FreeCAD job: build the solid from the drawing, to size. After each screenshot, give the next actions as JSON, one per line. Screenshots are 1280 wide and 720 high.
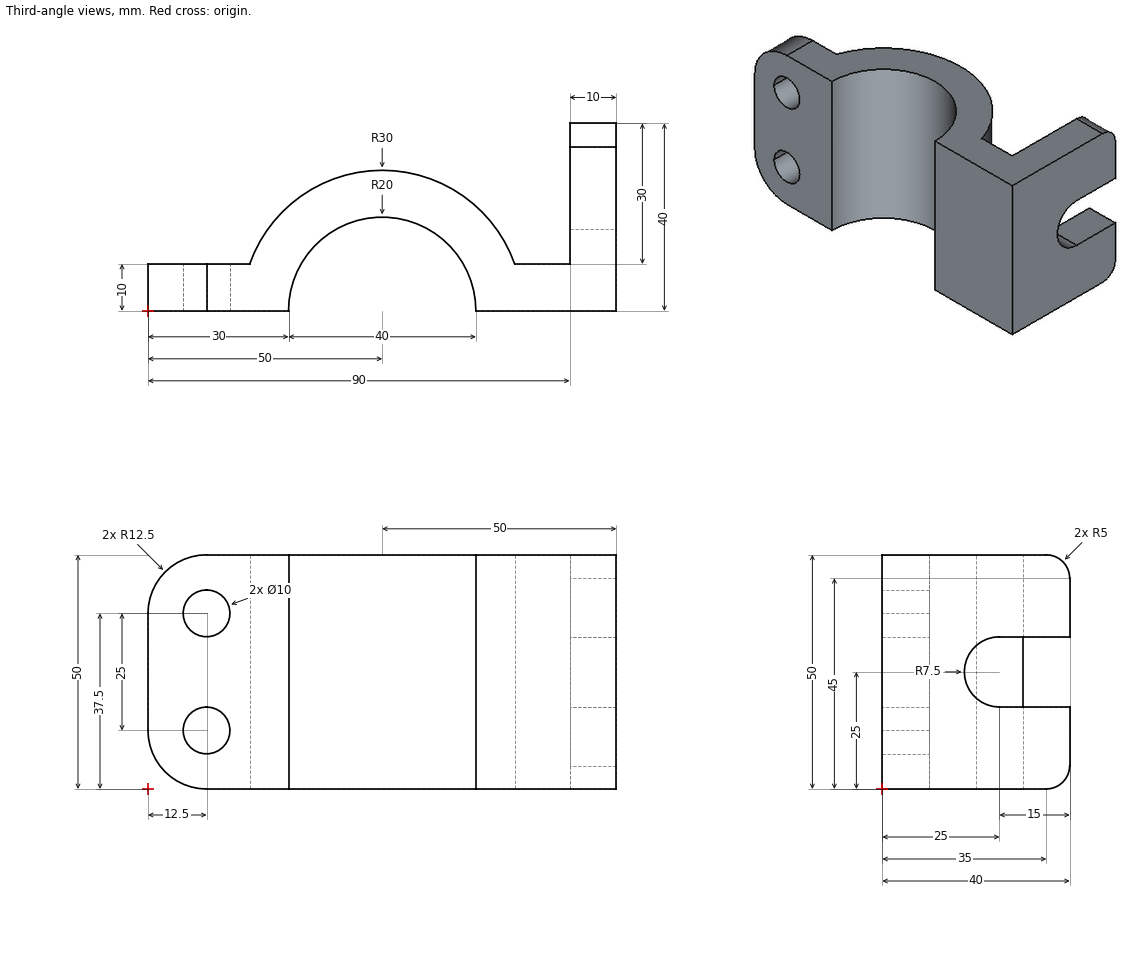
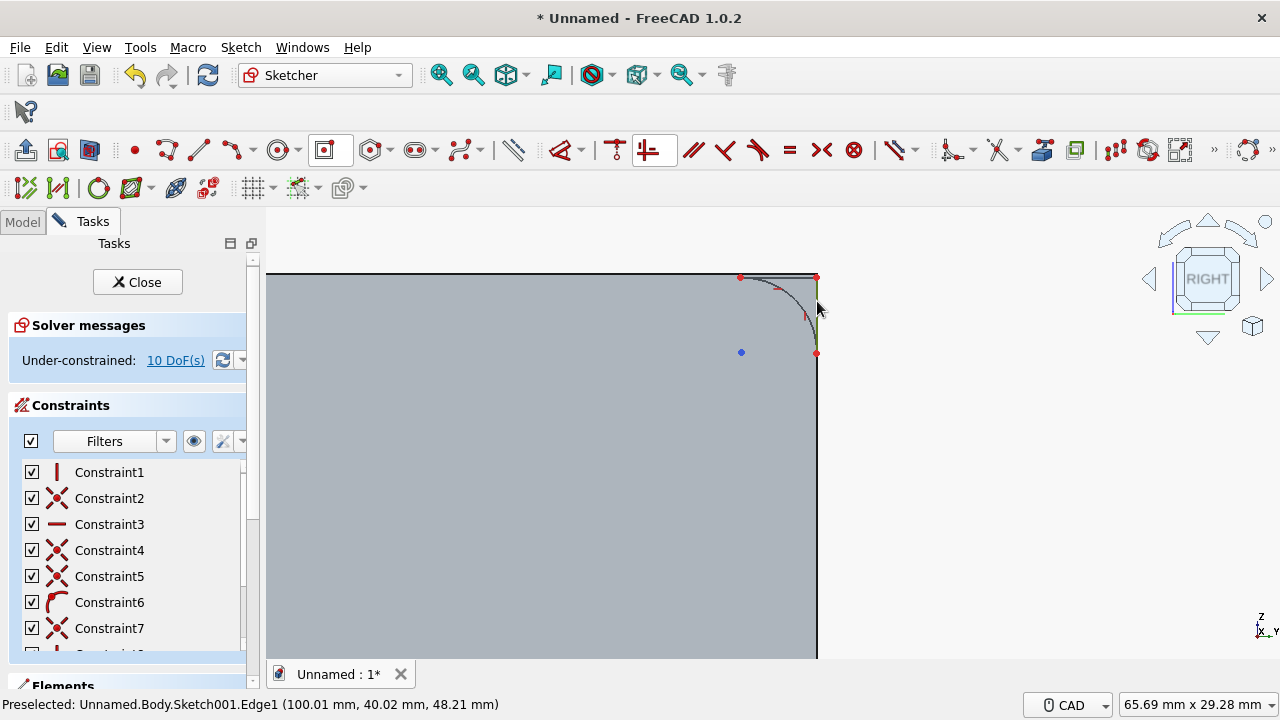
{"action": "left_click", "coordinate": [795, 300]}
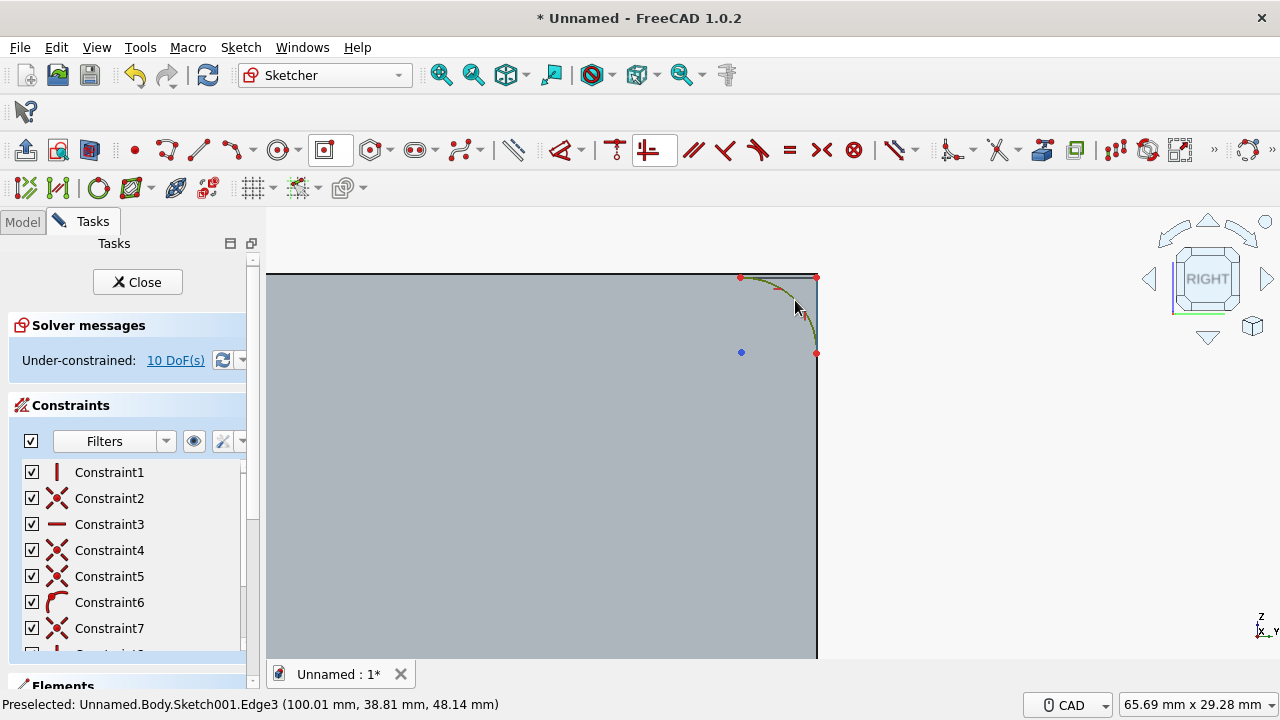
{"action": "left_click", "coordinate": [758, 150]}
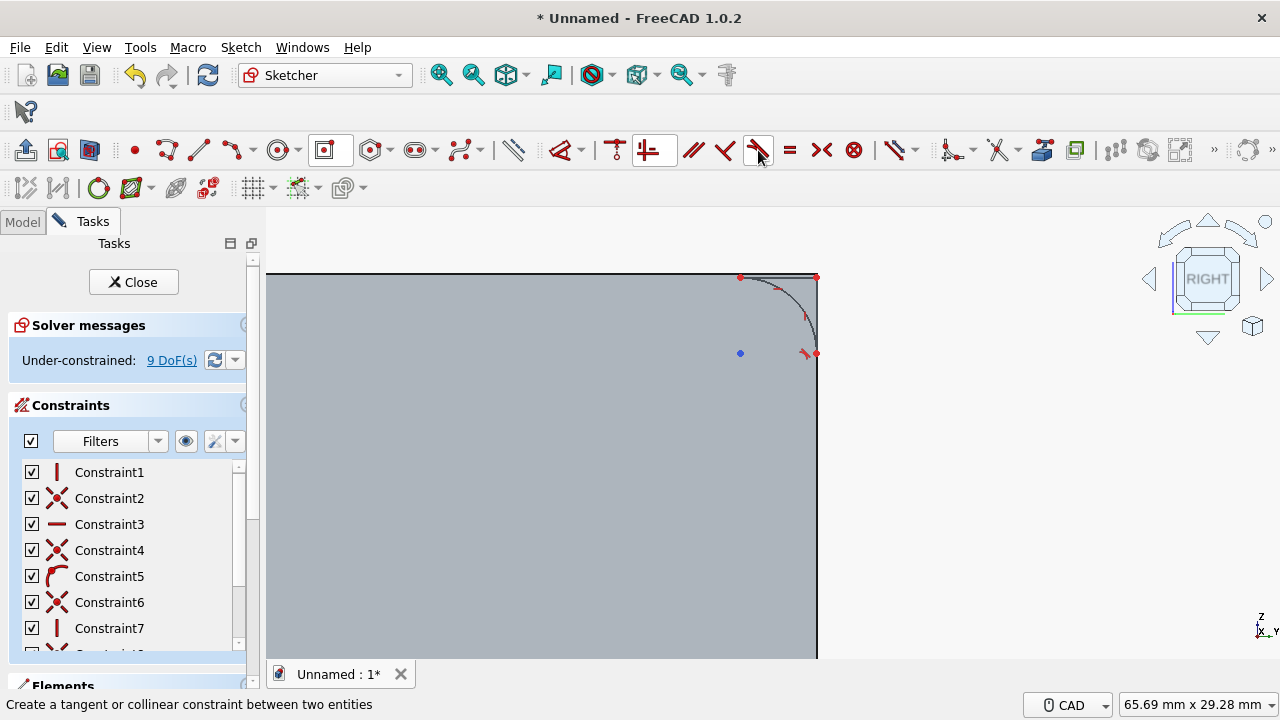
{"action": "left_click", "coordinate": [794, 278]}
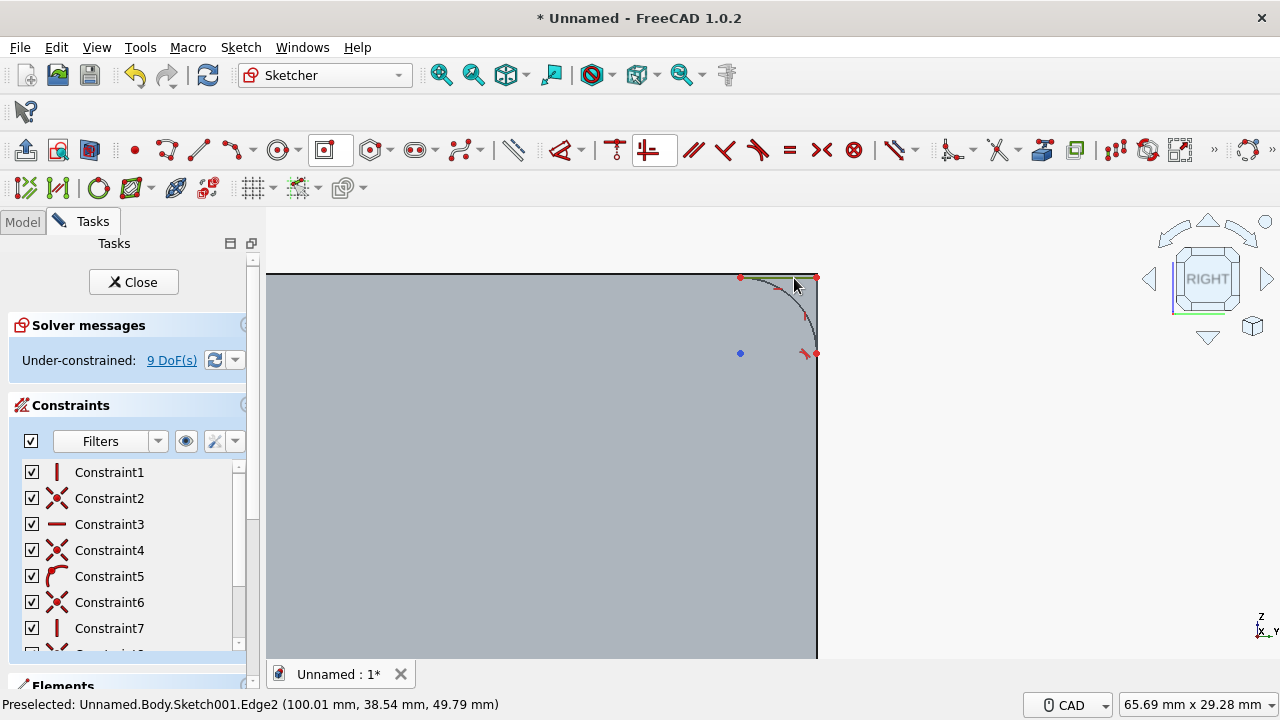
{"action": "left_click", "coordinate": [795, 300]}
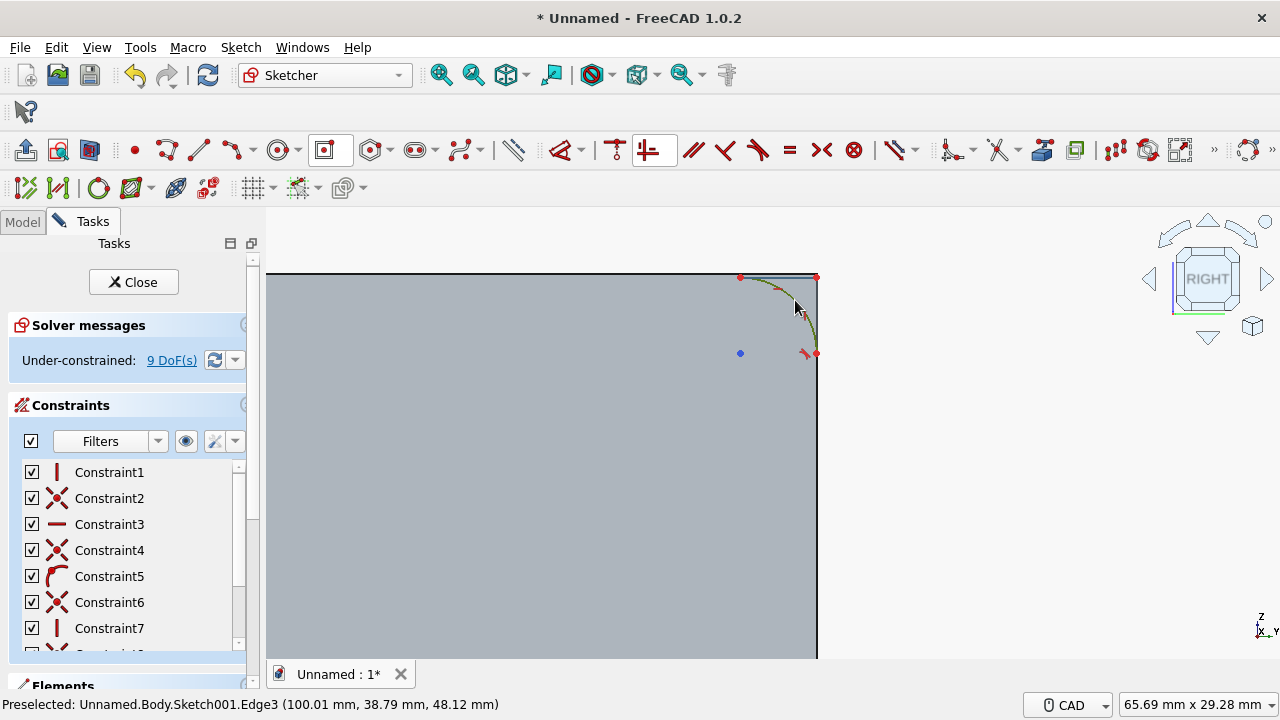
{"action": "left_click", "coordinate": [758, 150]}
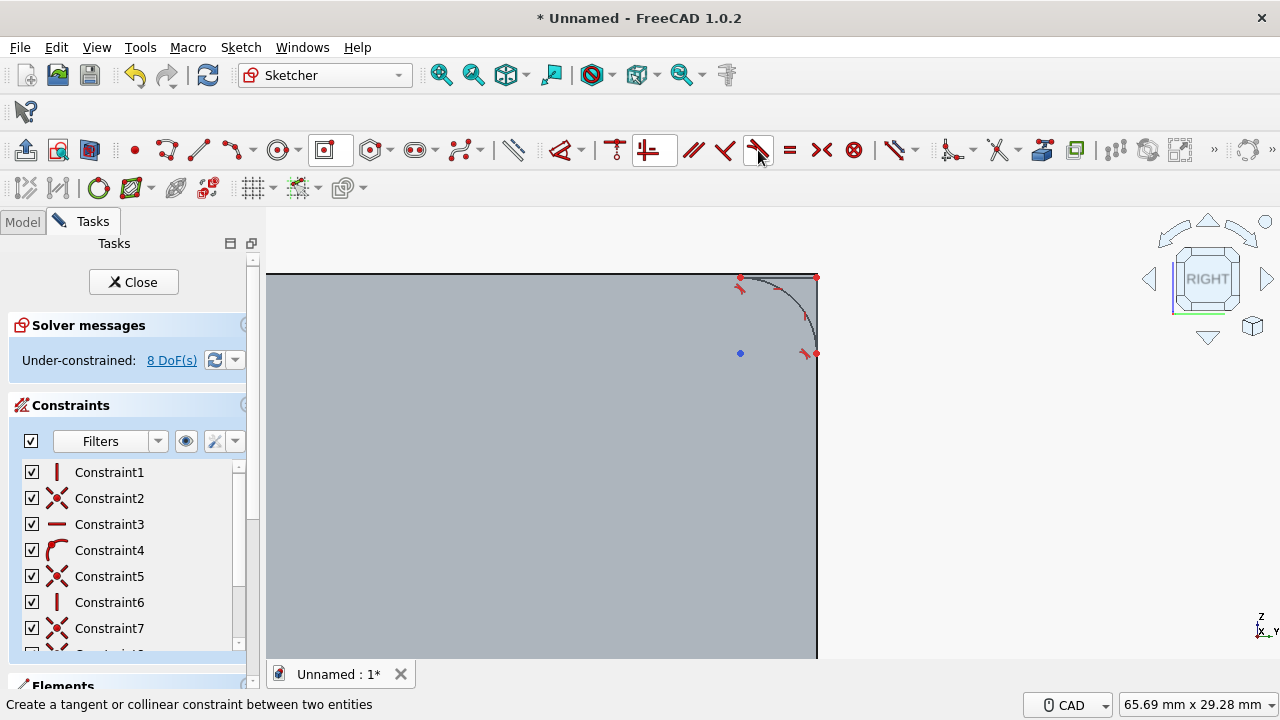
{"action": "scroll", "coordinate": [819, 301], "scroll_direction": "down", "scroll_amount": 5}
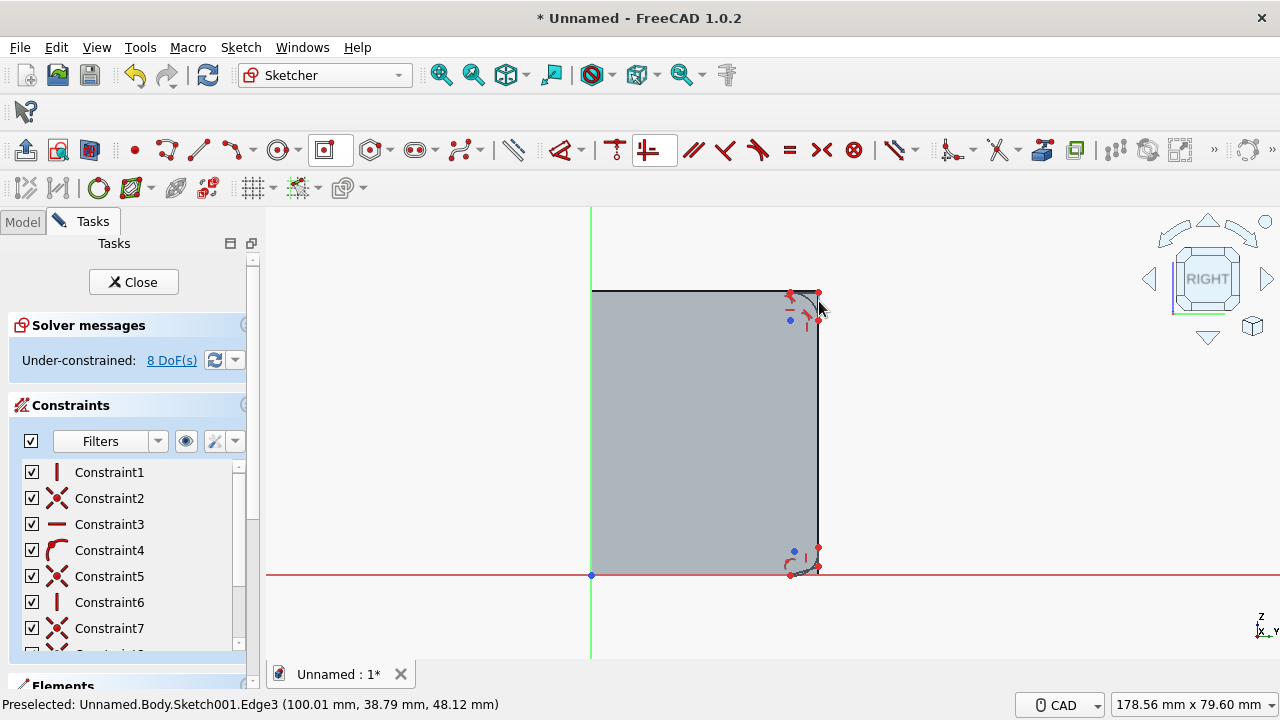
{"action": "scroll", "coordinate": [801, 572], "scroll_direction": "up", "scroll_amount": 9}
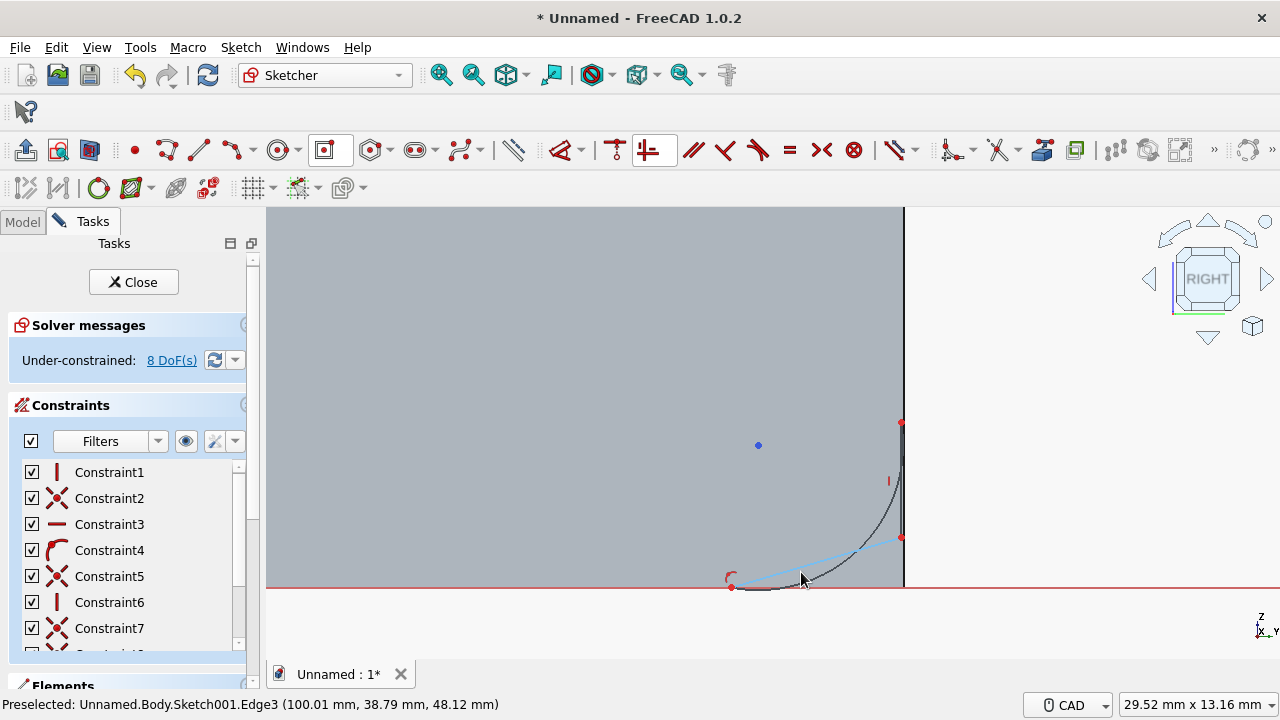
{"action": "left_click", "coordinate": [800, 568]}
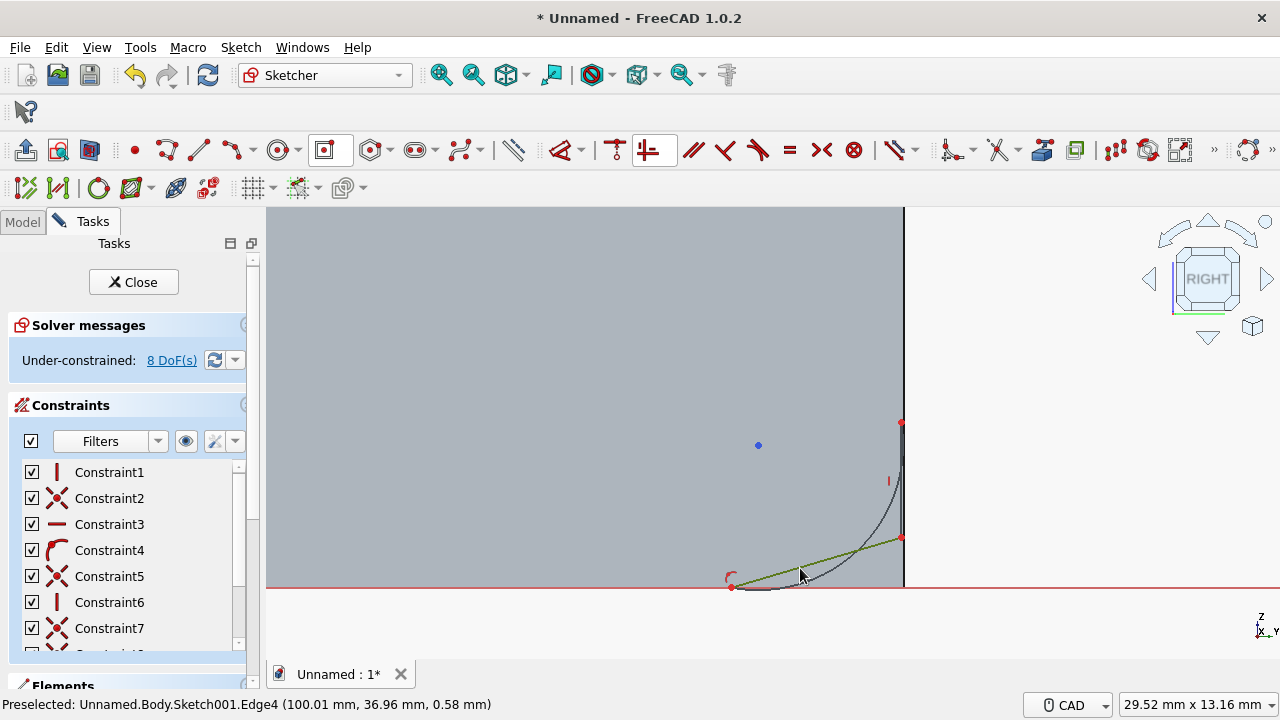
{"action": "scroll", "coordinate": [891, 504], "scroll_direction": "up", "scroll_amount": 2}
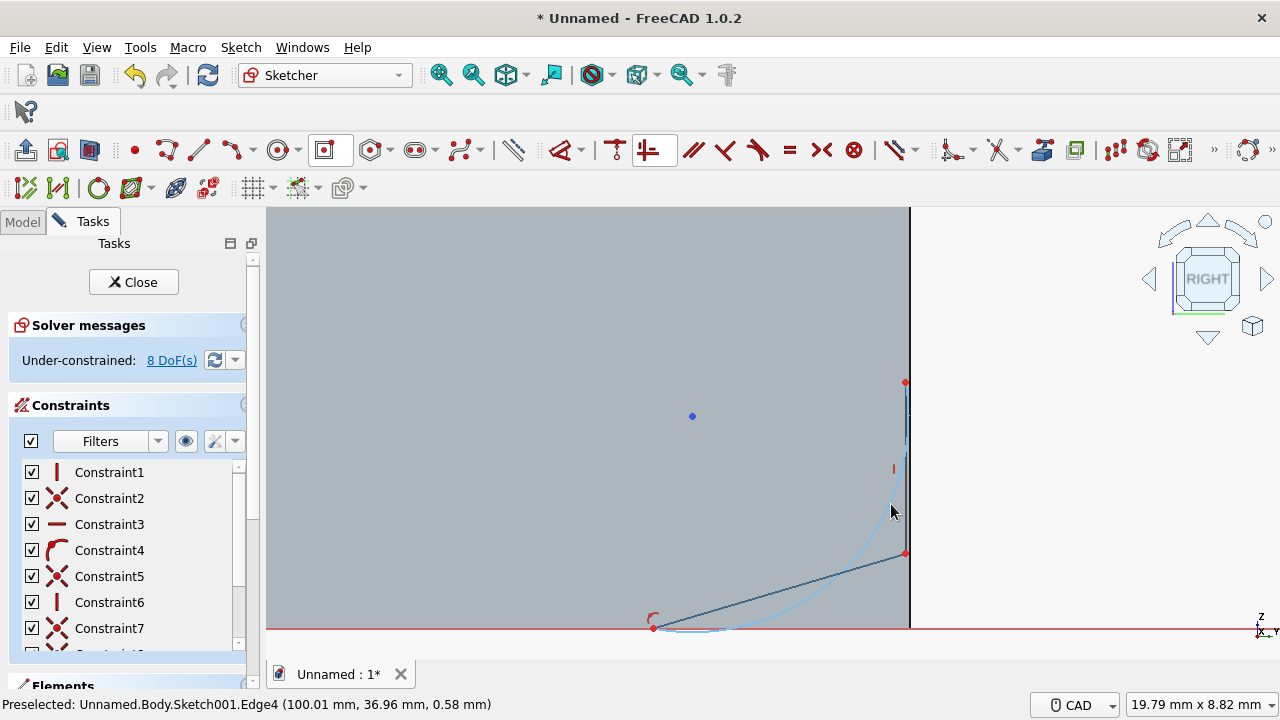
{"action": "left_click", "coordinate": [890, 504]}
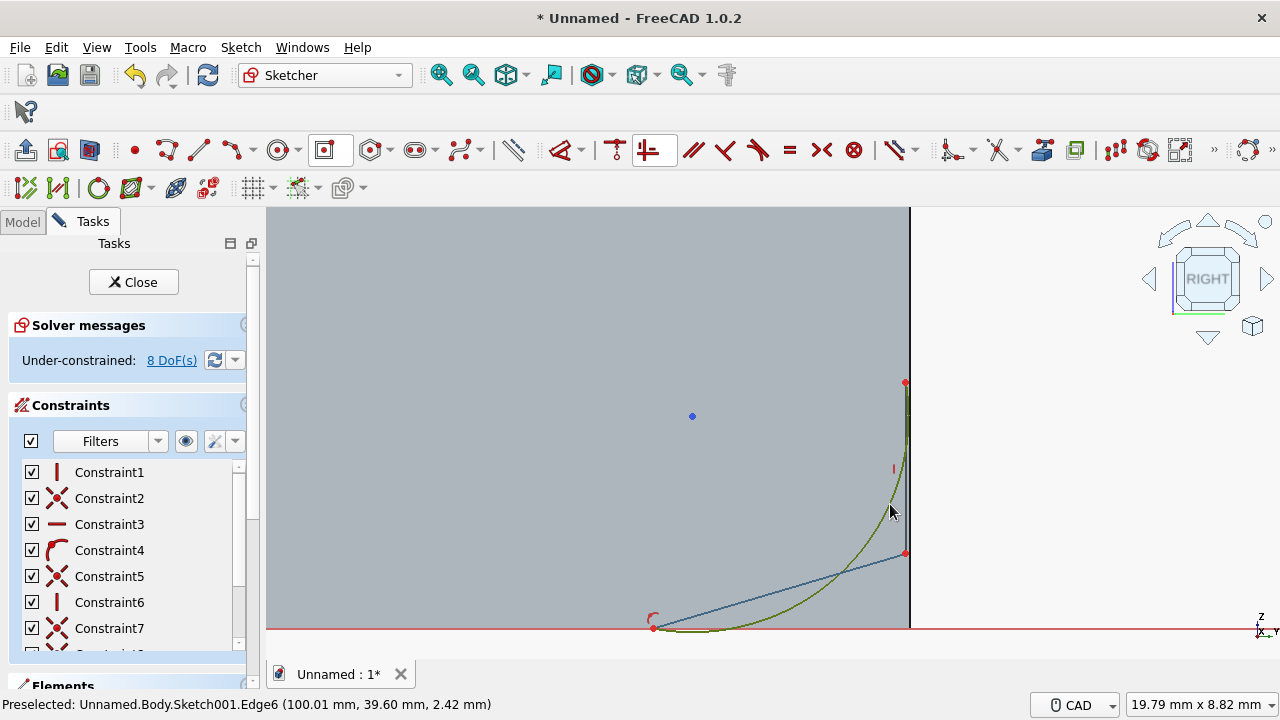
{"action": "left_click", "coordinate": [758, 150]}